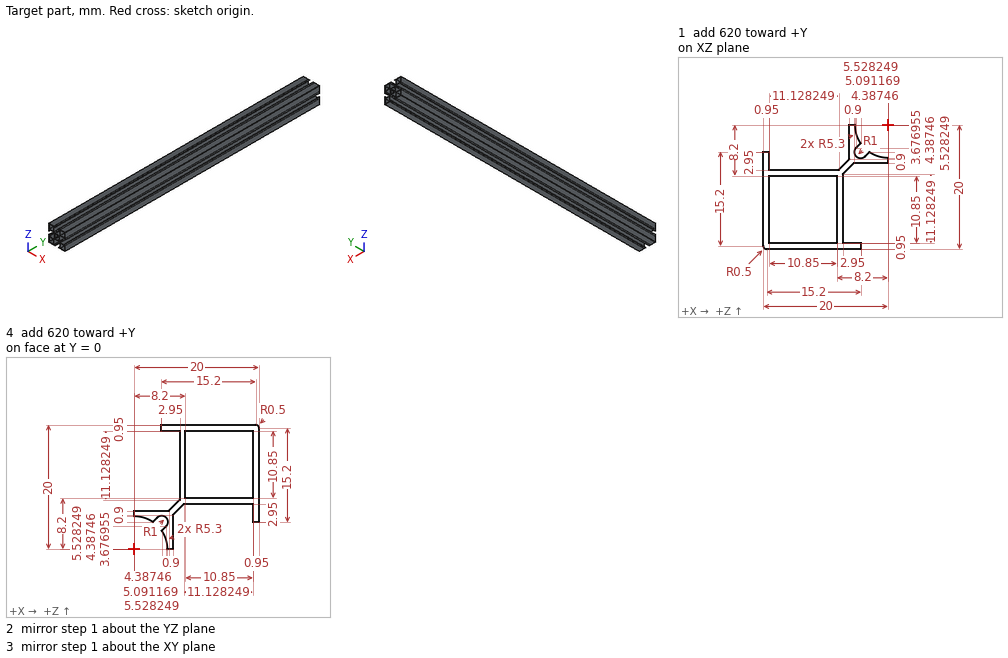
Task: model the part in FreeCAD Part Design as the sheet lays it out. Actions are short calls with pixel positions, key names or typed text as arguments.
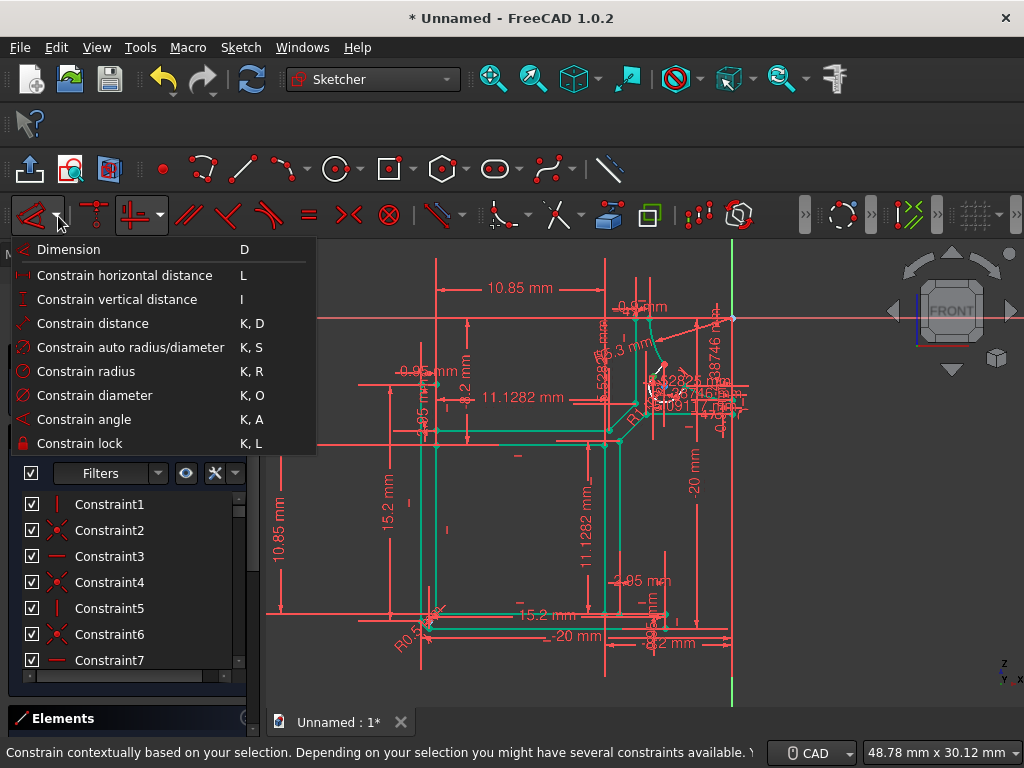
click(164, 299)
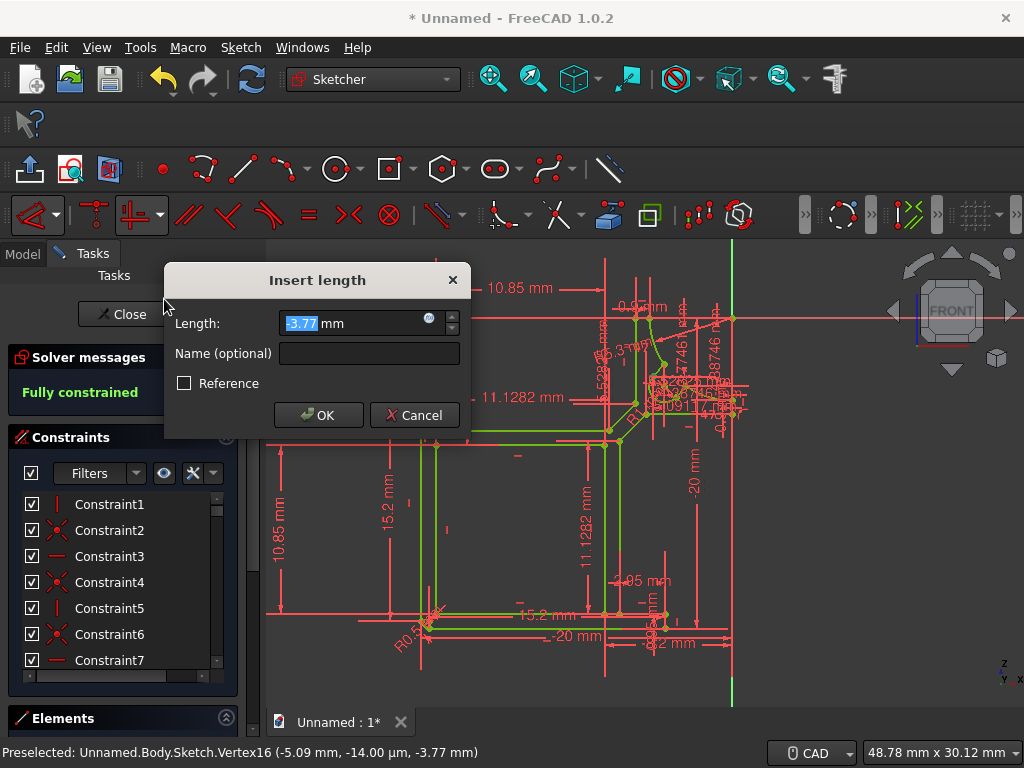
text(-3.676955)
key(Return)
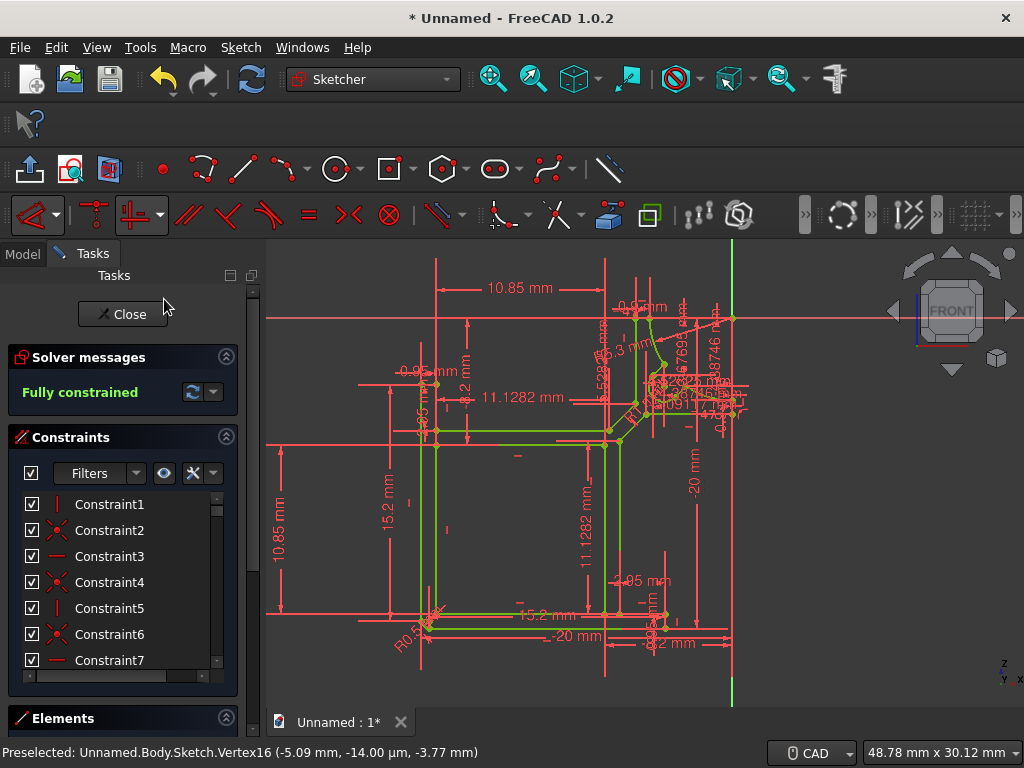
click(123, 314)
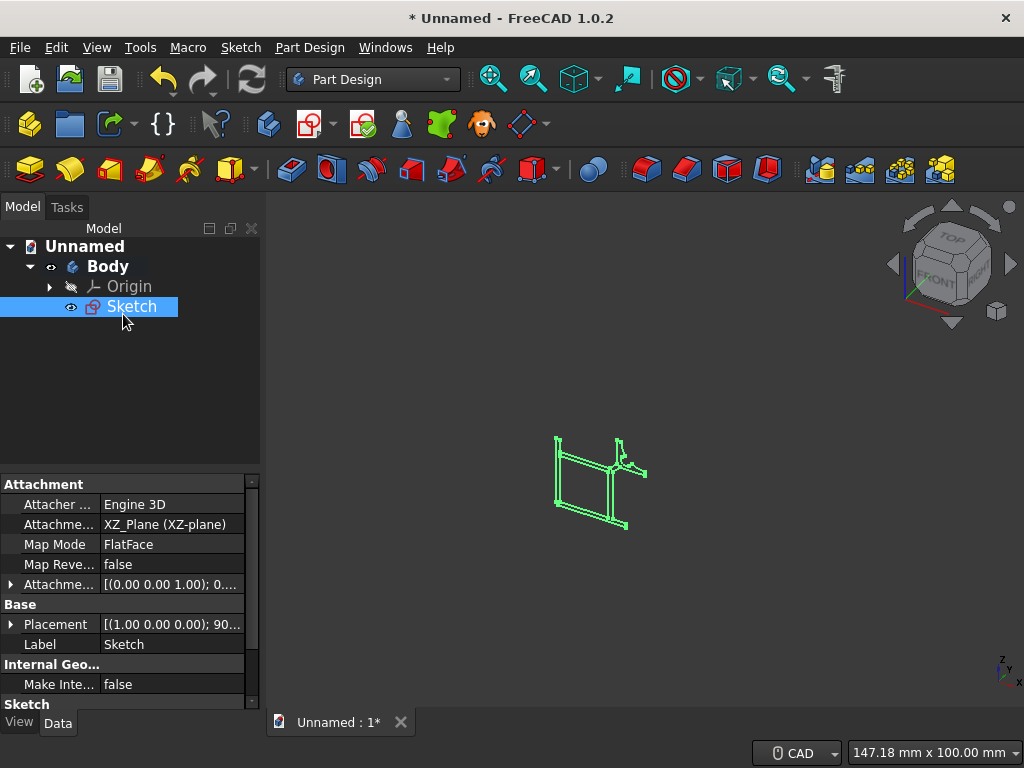
click(30, 170)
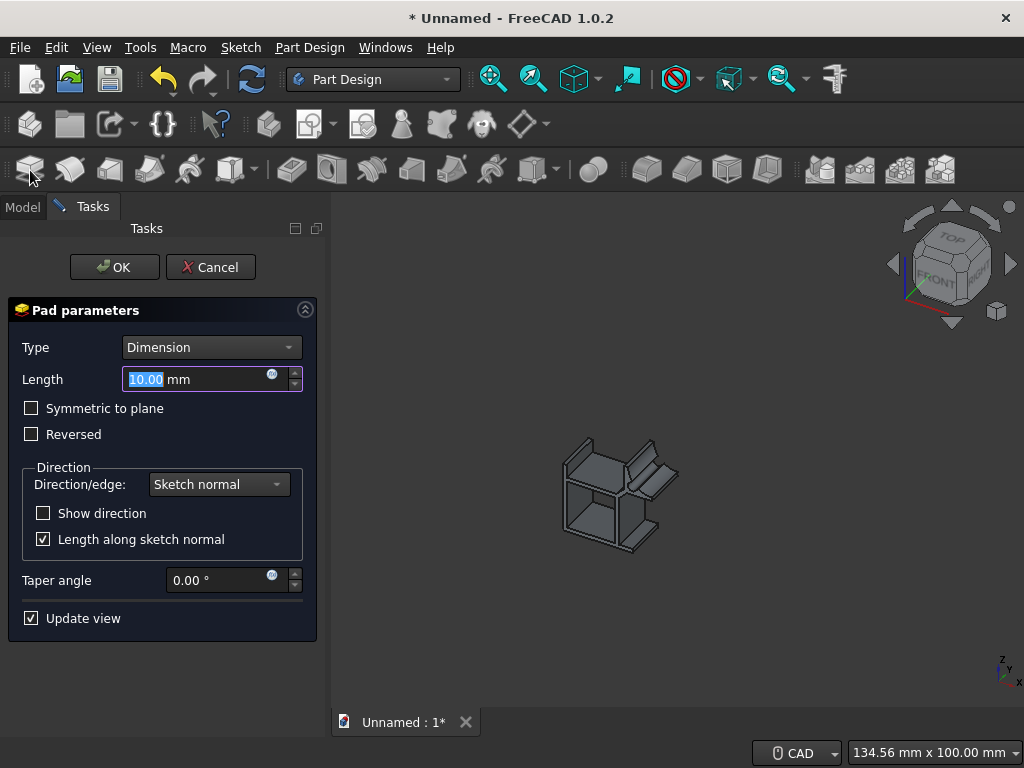
text(620)
key(Tab)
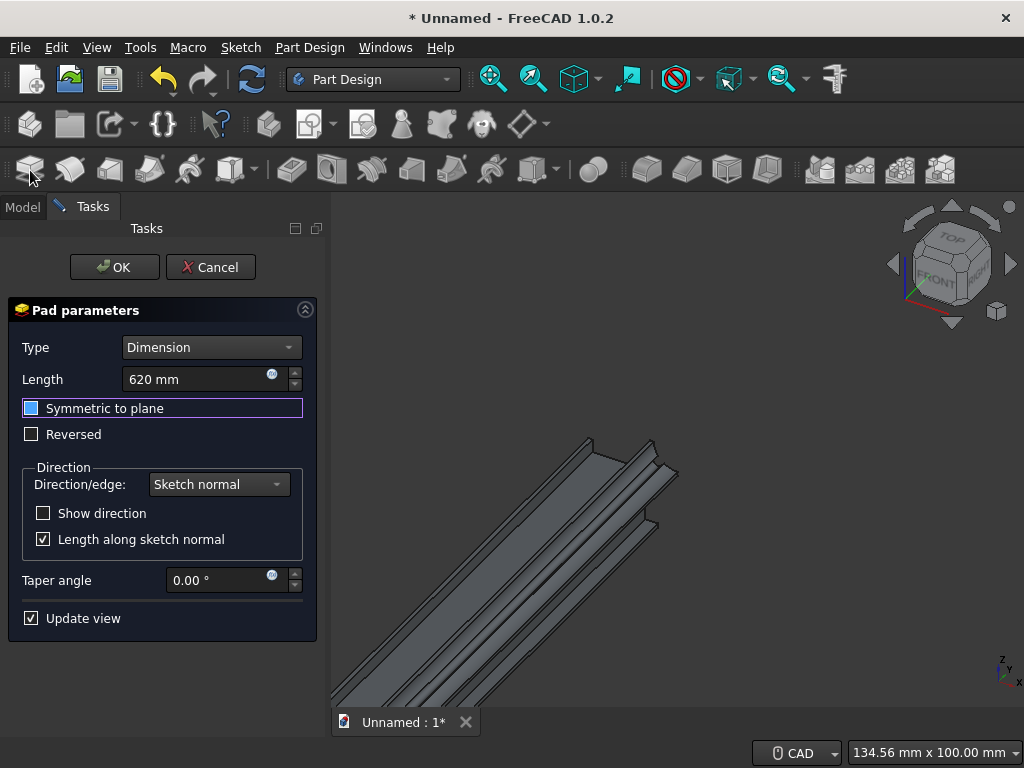
click(30, 434)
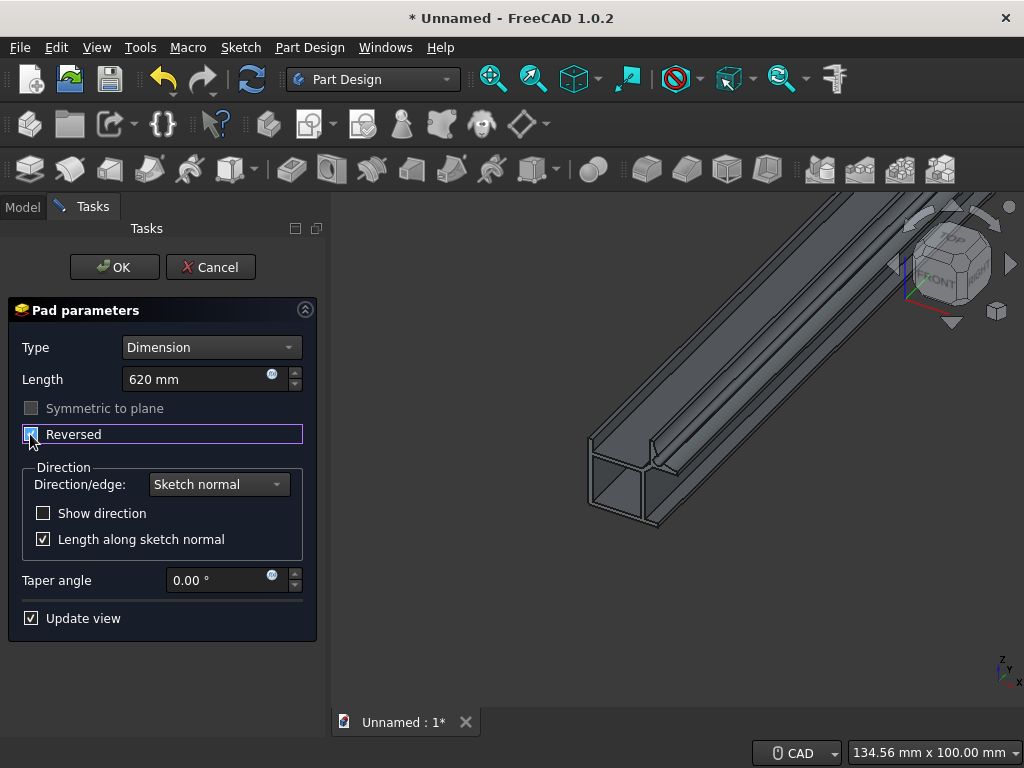
click(115, 267)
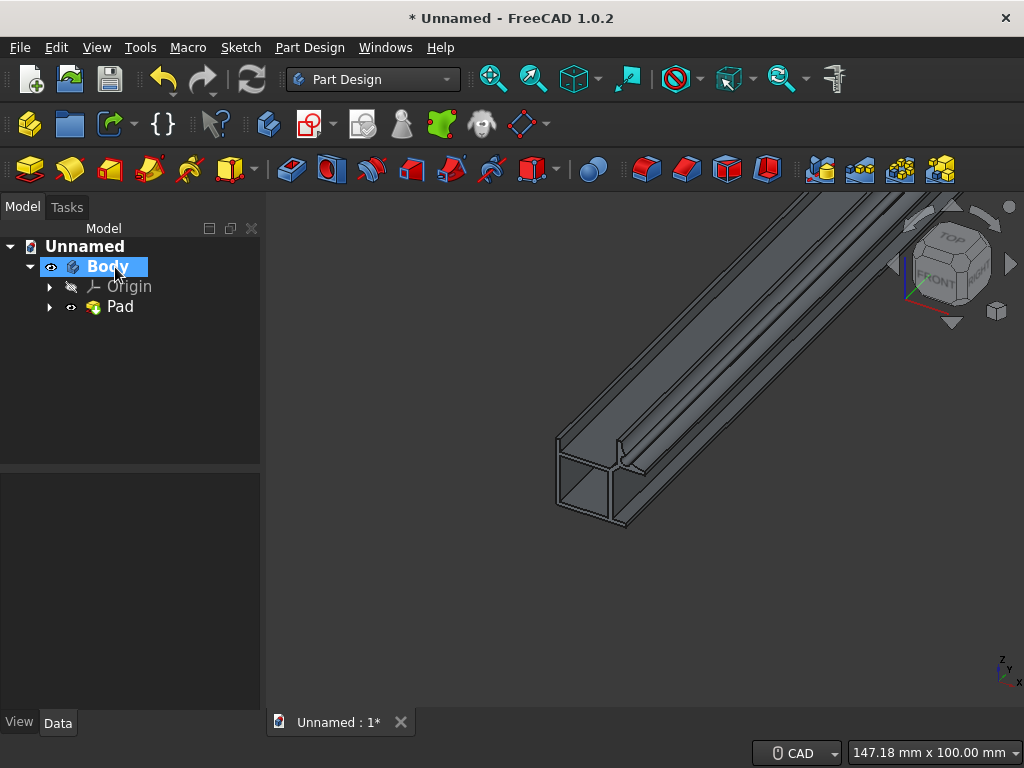
click(494, 80)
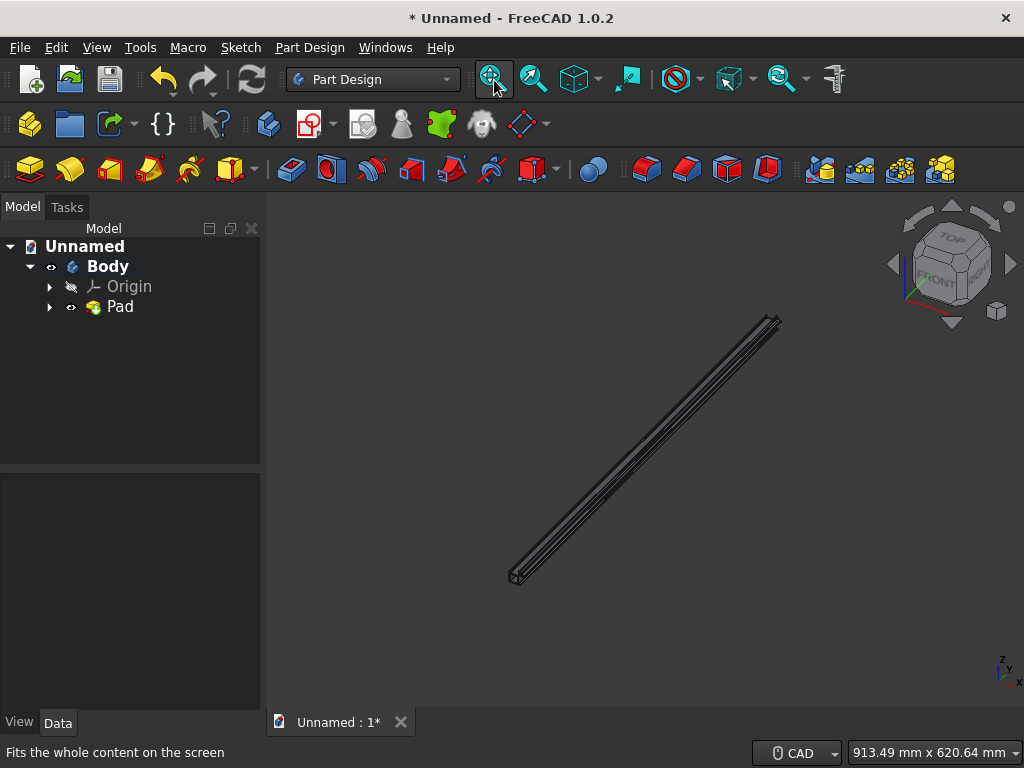
click(116, 307)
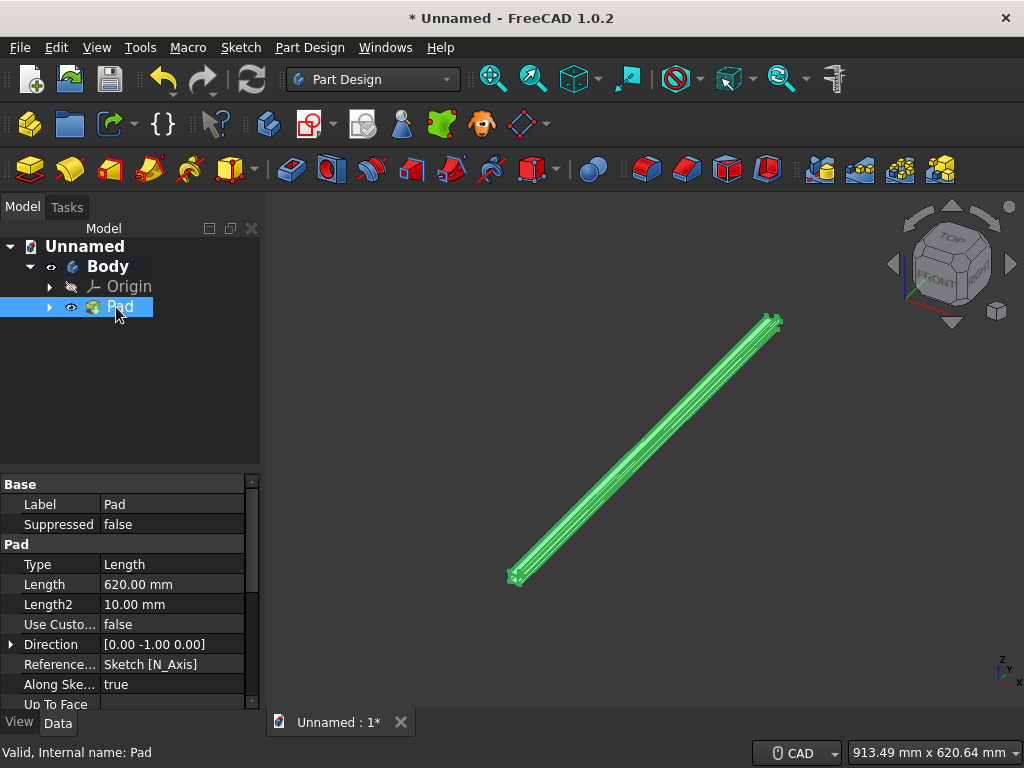
click(820, 170)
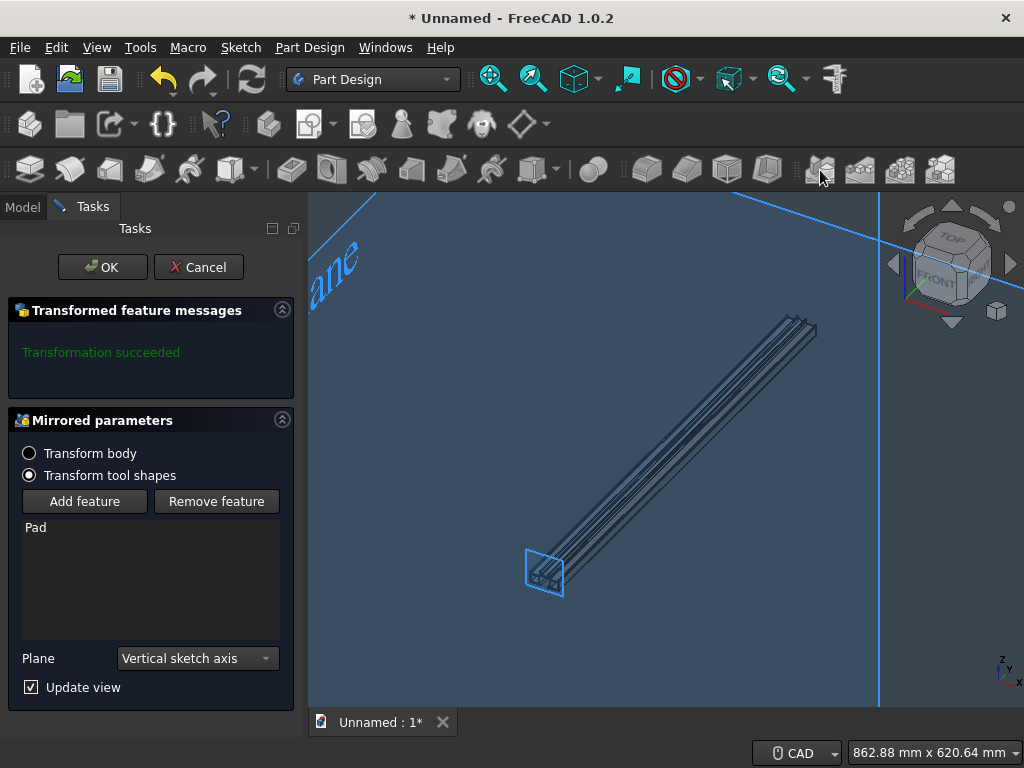
click(198, 658)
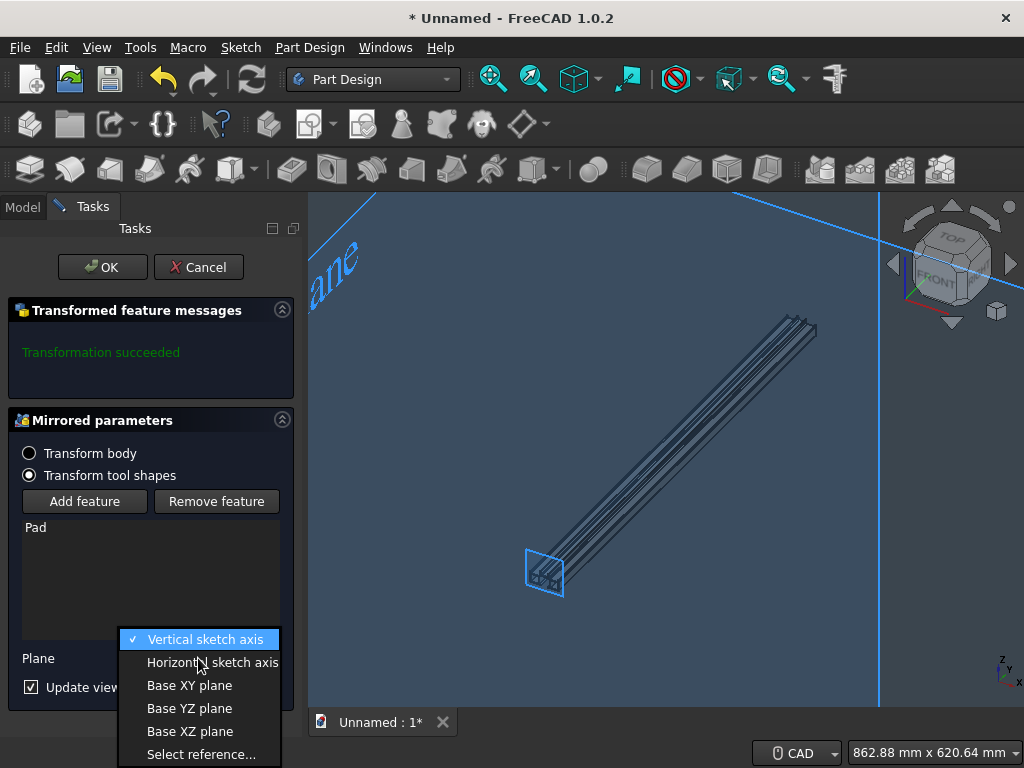
click(198, 708)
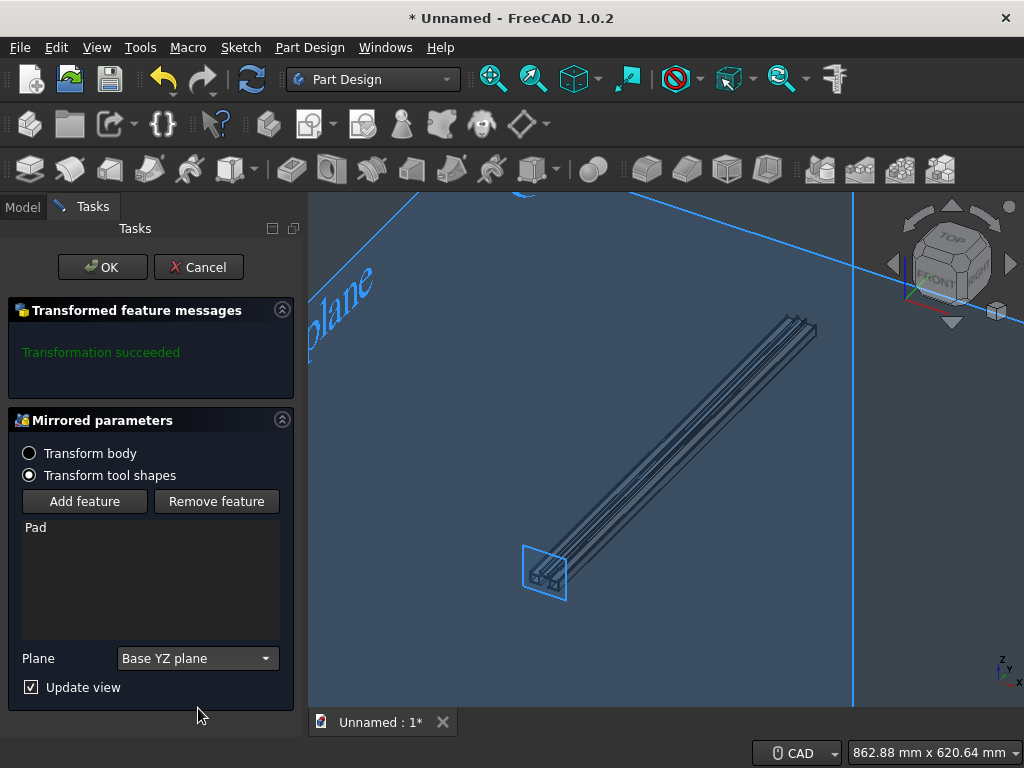
click(103, 267)